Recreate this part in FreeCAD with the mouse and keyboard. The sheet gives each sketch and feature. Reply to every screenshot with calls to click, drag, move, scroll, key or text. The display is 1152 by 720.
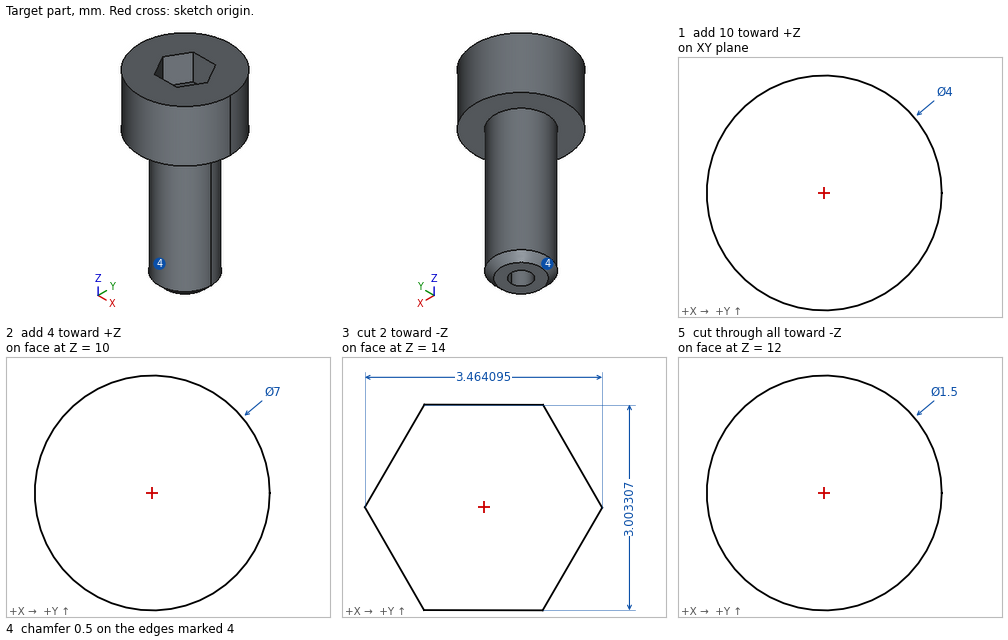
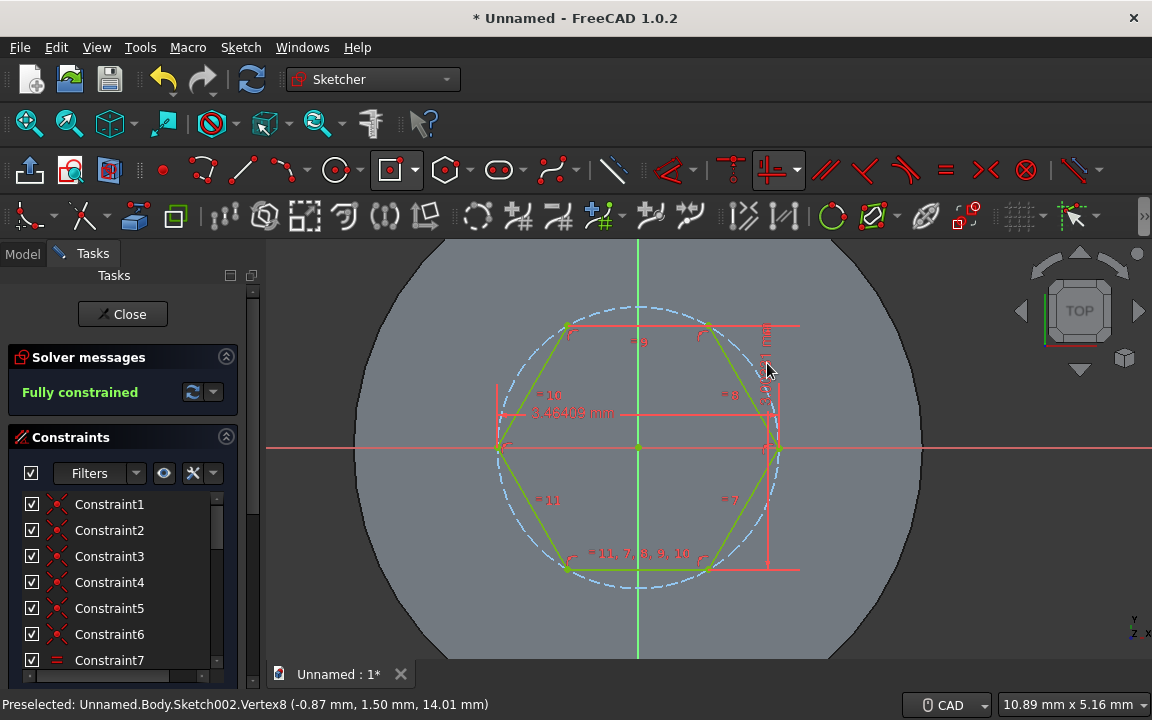
click(123, 314)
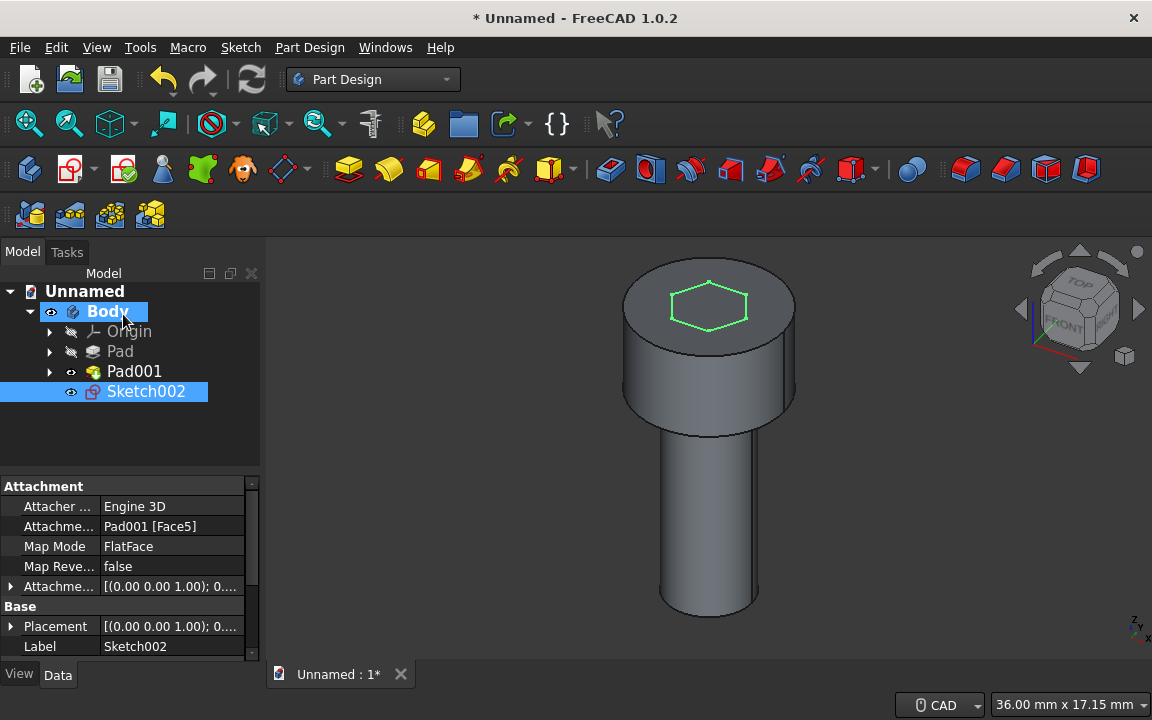
click(612, 170)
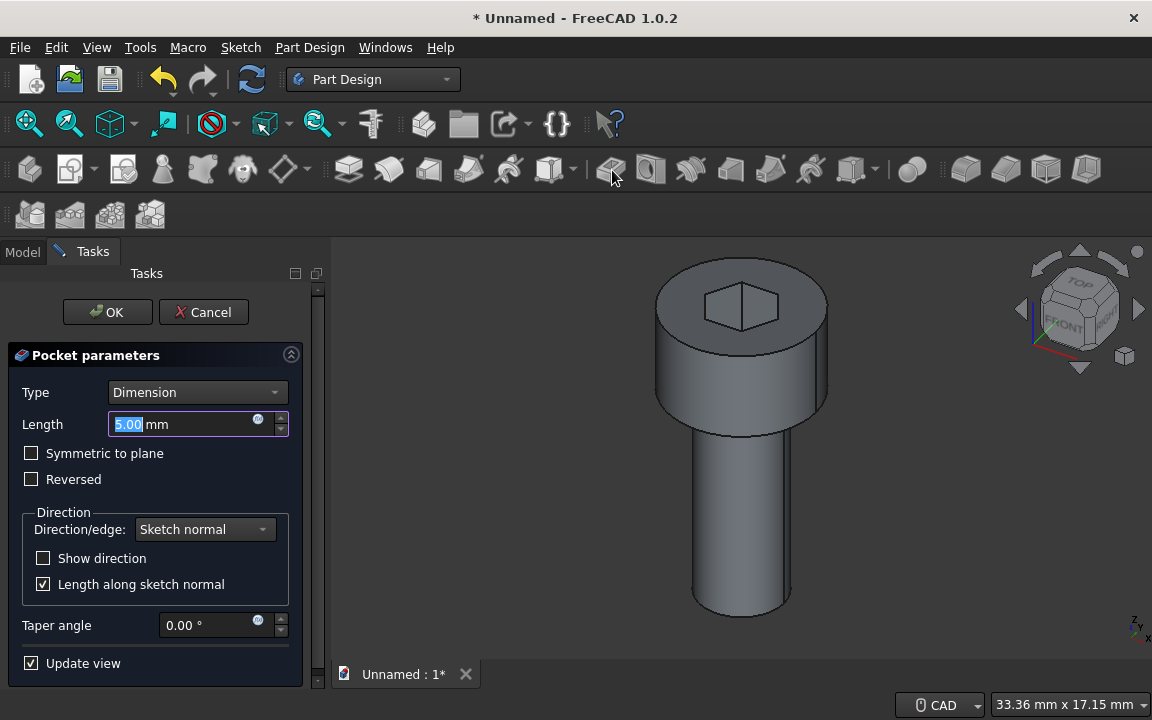
text(2)
key(Tab)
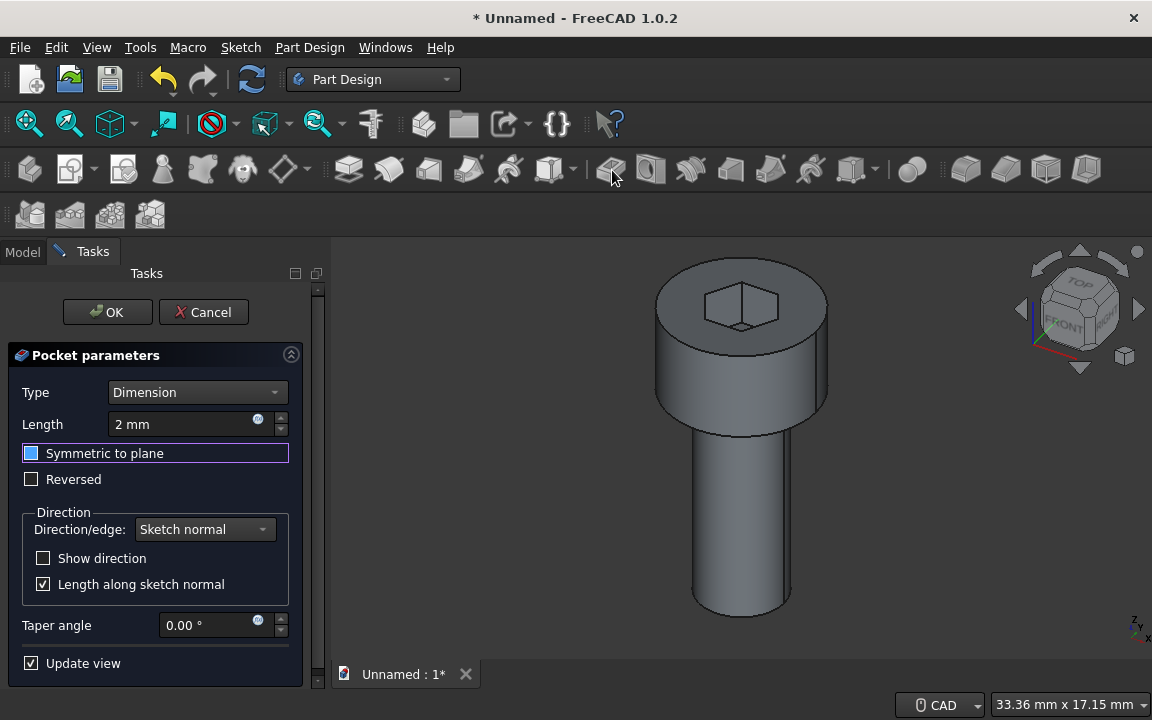
click(108, 312)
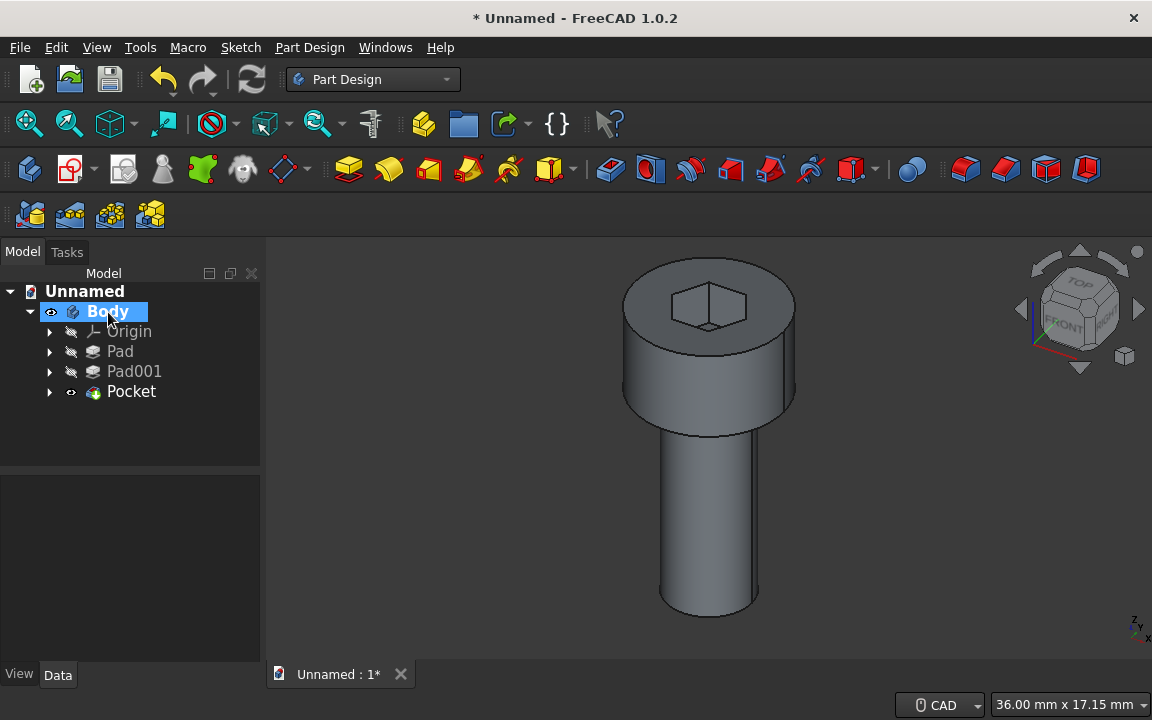
key(0)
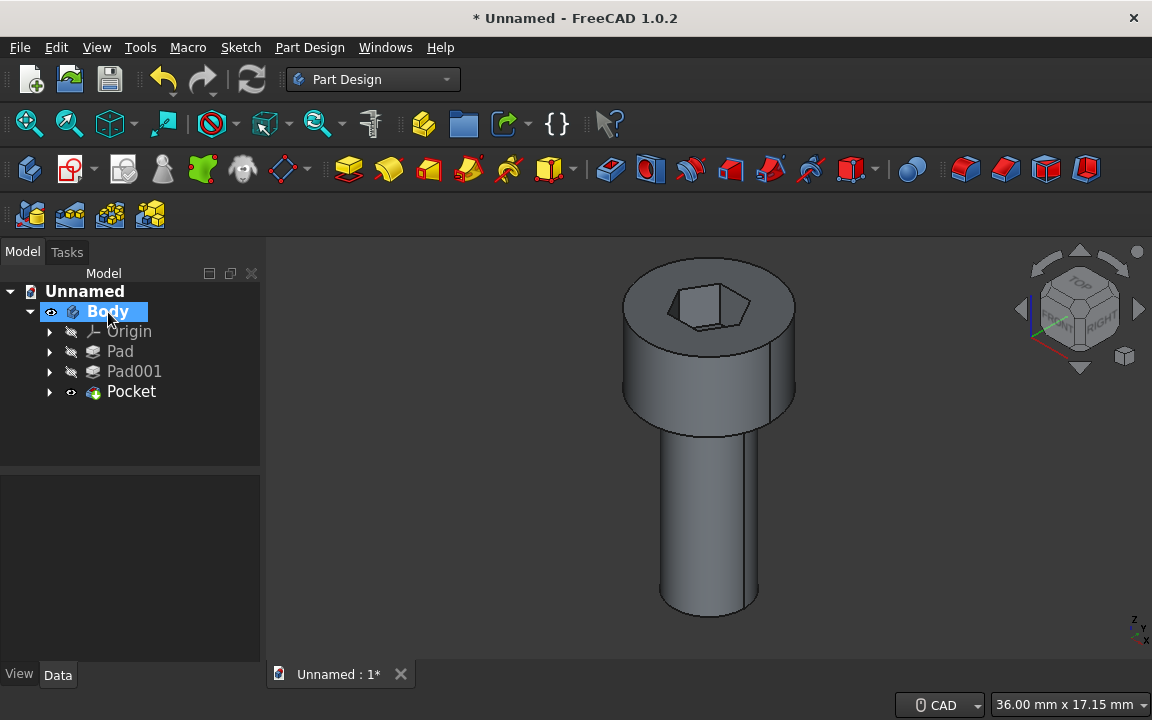
click(30, 124)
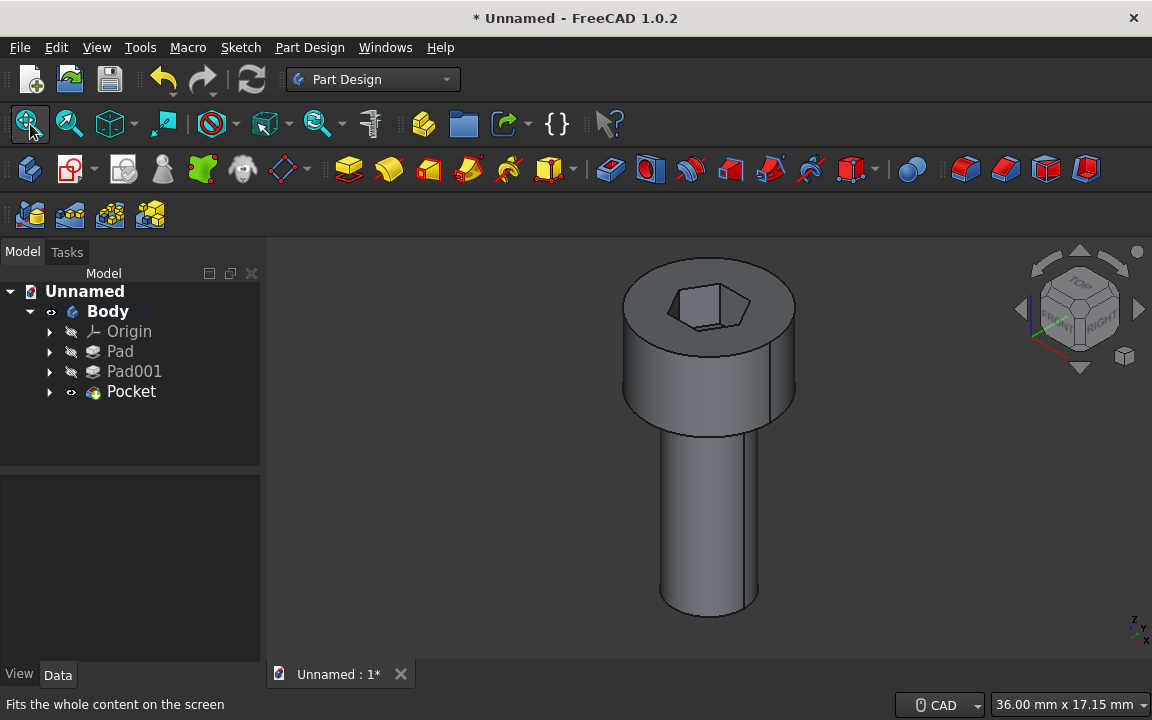
key(2)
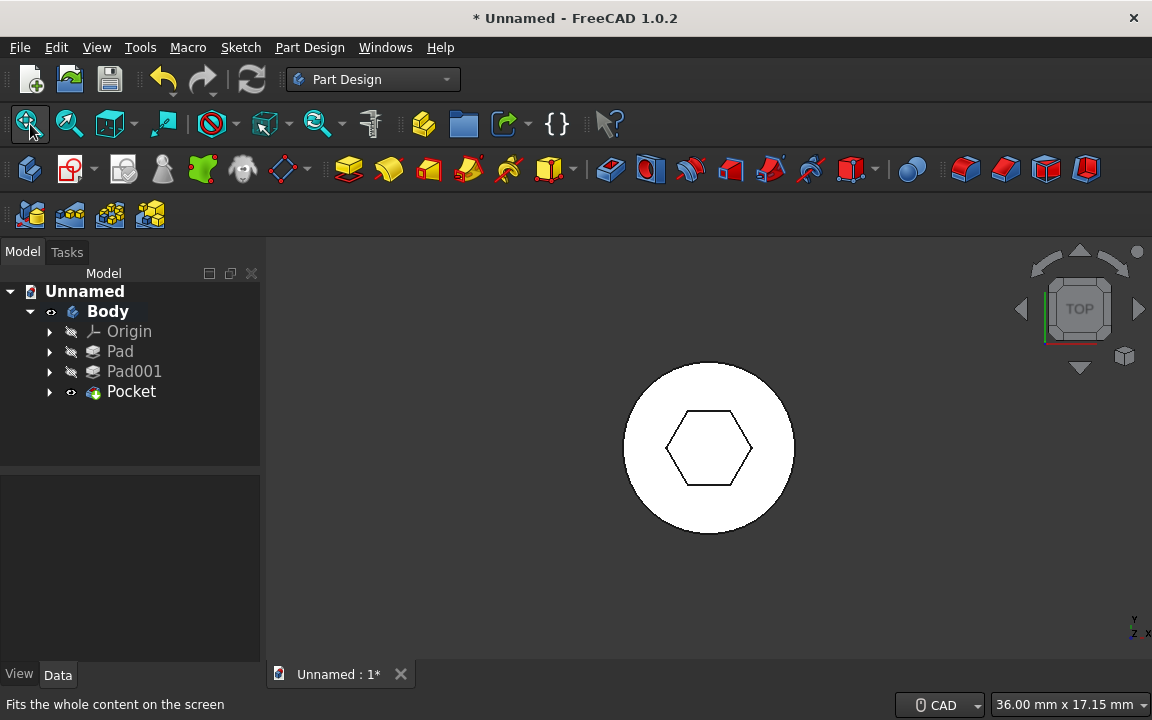
click(30, 124)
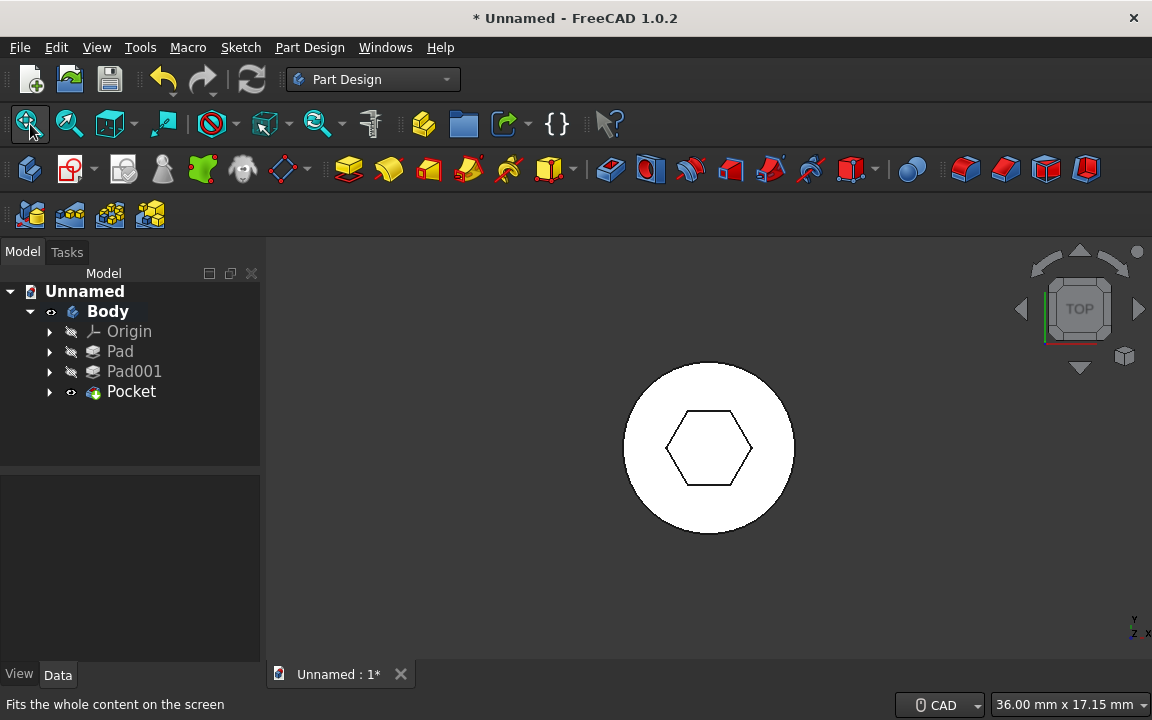
key(1)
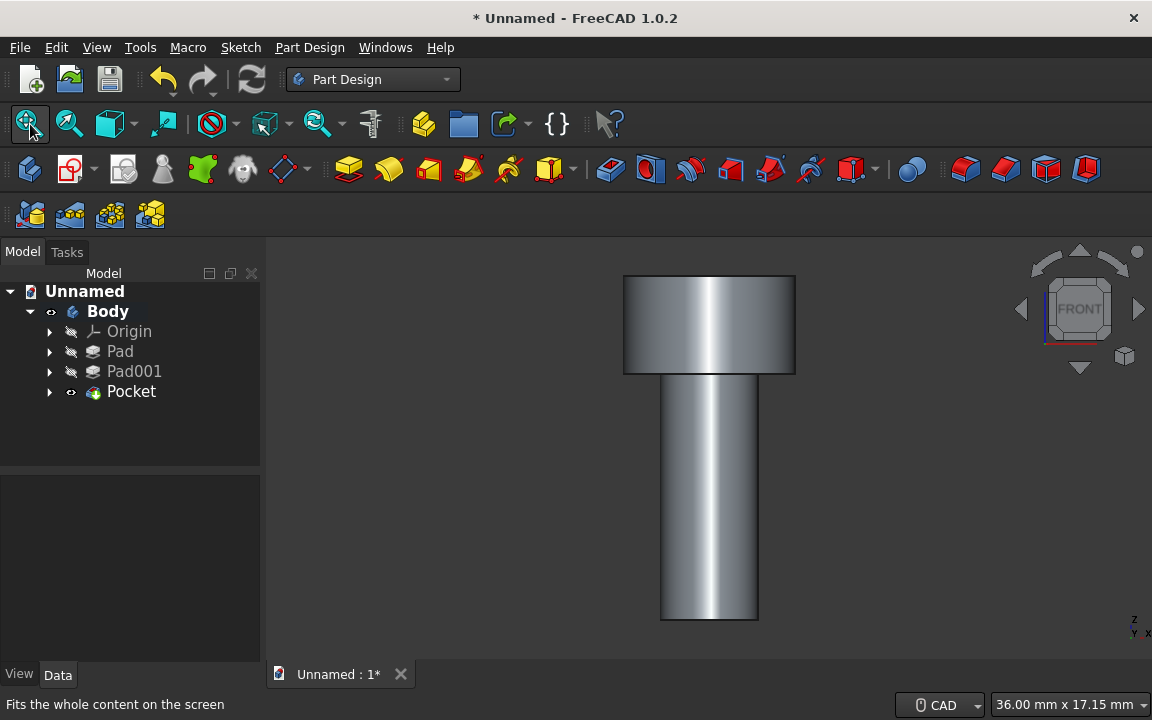
click(669, 619)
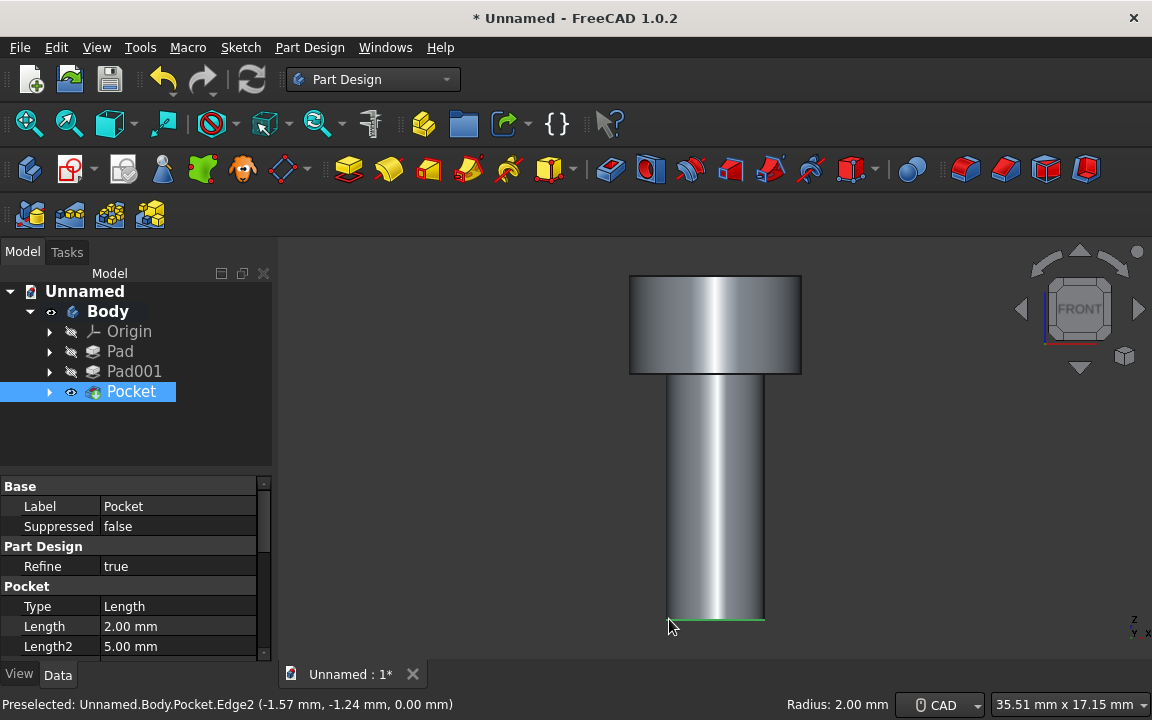
click(1006, 170)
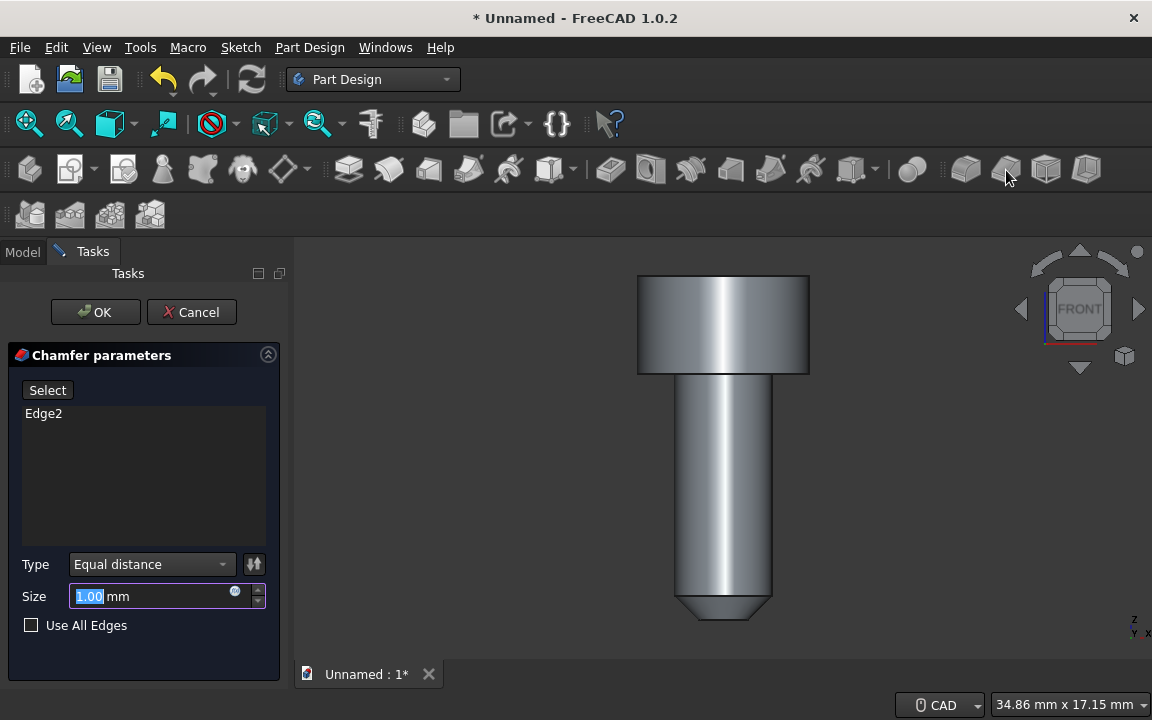
text(0.5)
key(Tab)